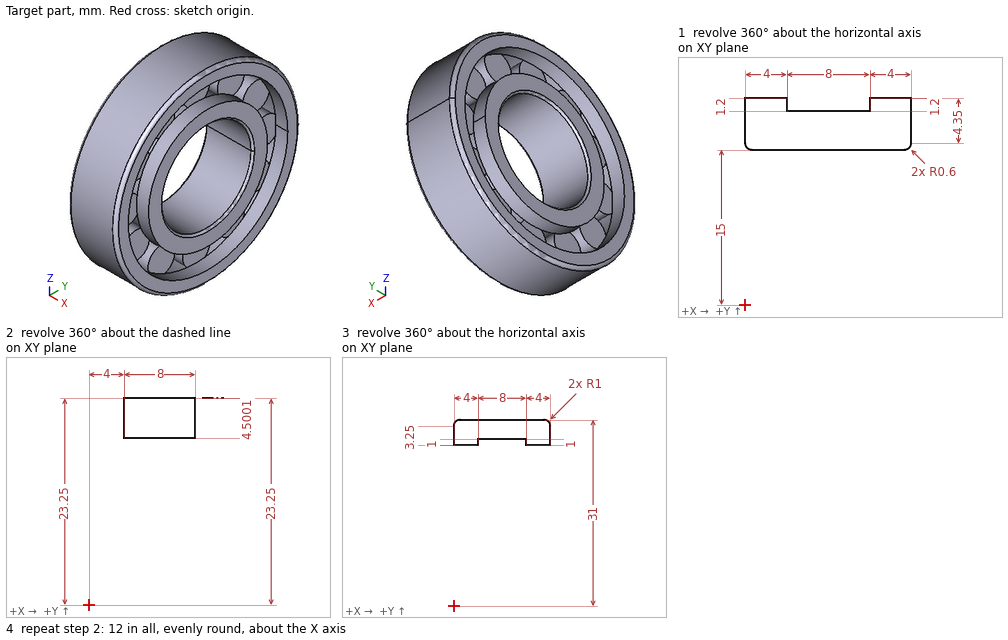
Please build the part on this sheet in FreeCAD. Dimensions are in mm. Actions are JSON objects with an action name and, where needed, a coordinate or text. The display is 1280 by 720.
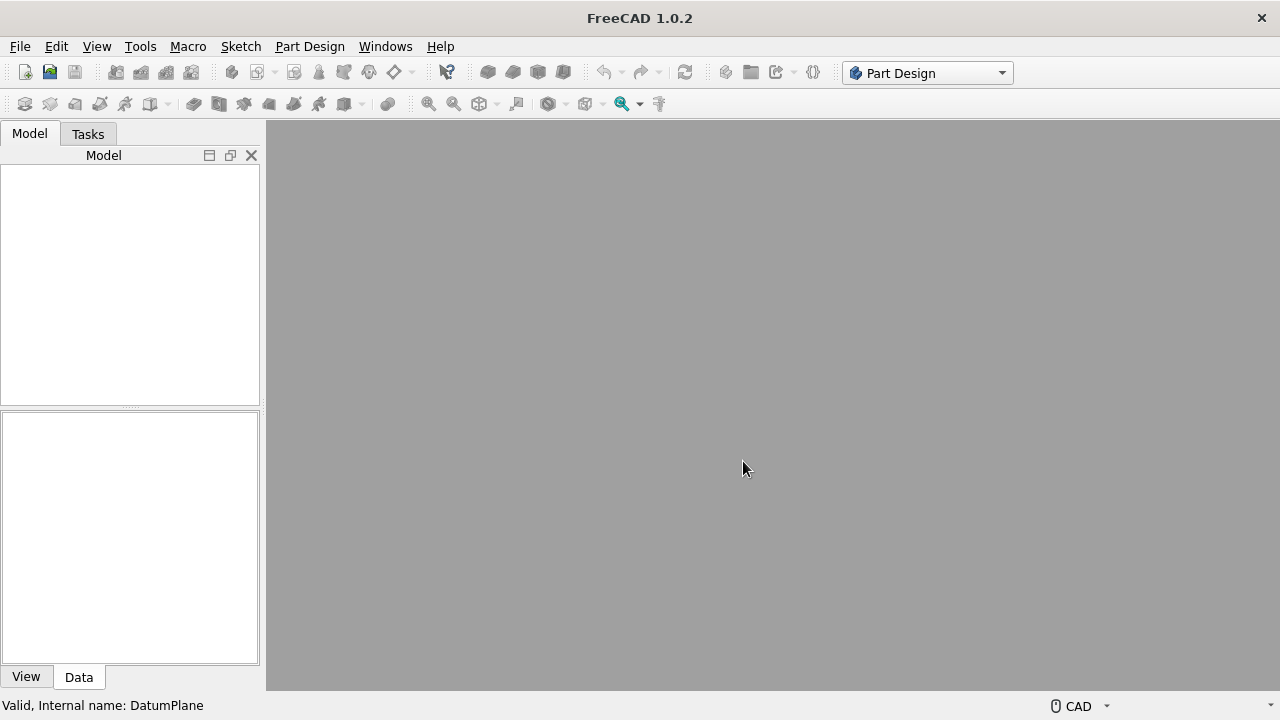
{"action": "left_click", "coordinate": [25, 72]}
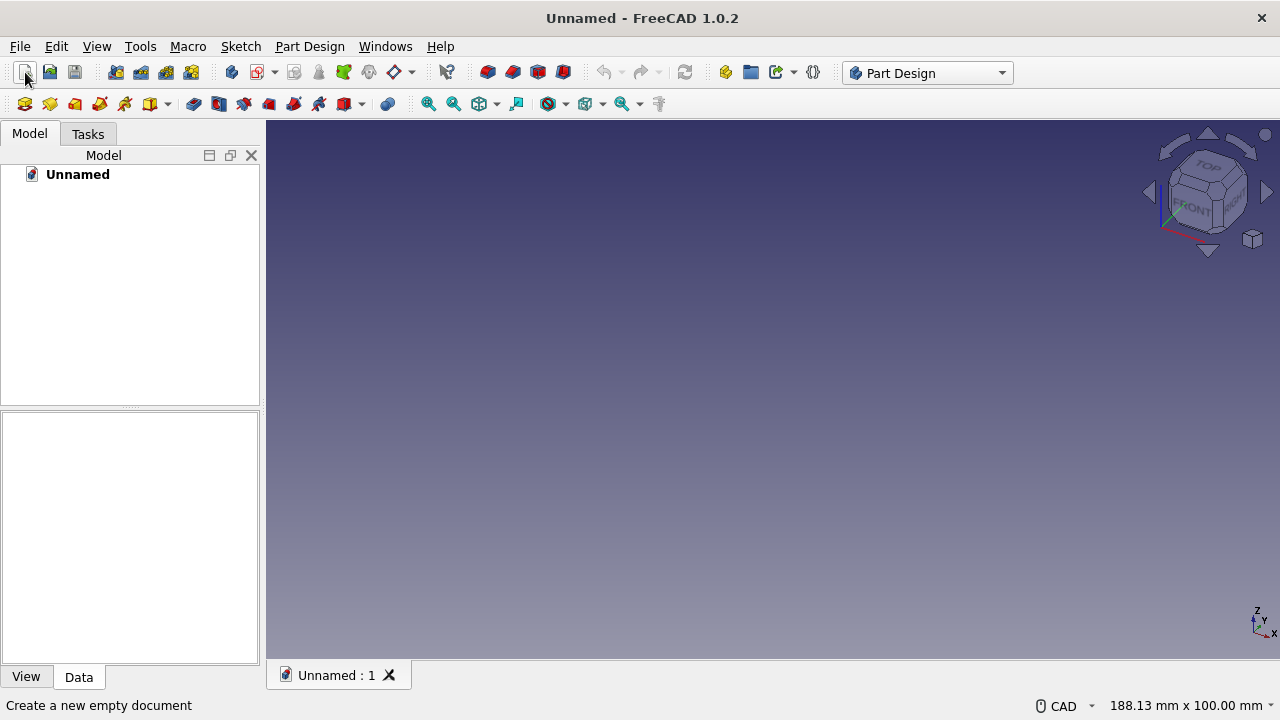
{"action": "left_click", "coordinate": [256, 72]}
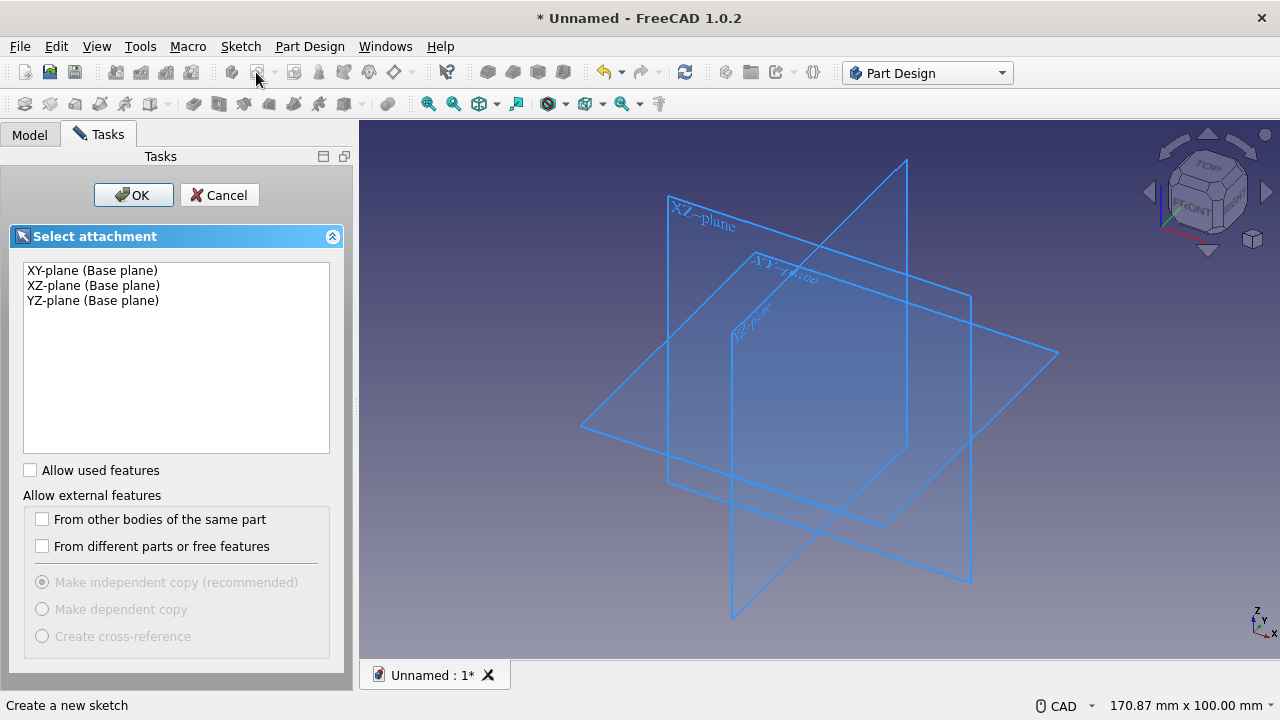
{"action": "left_click", "coordinate": [84, 270]}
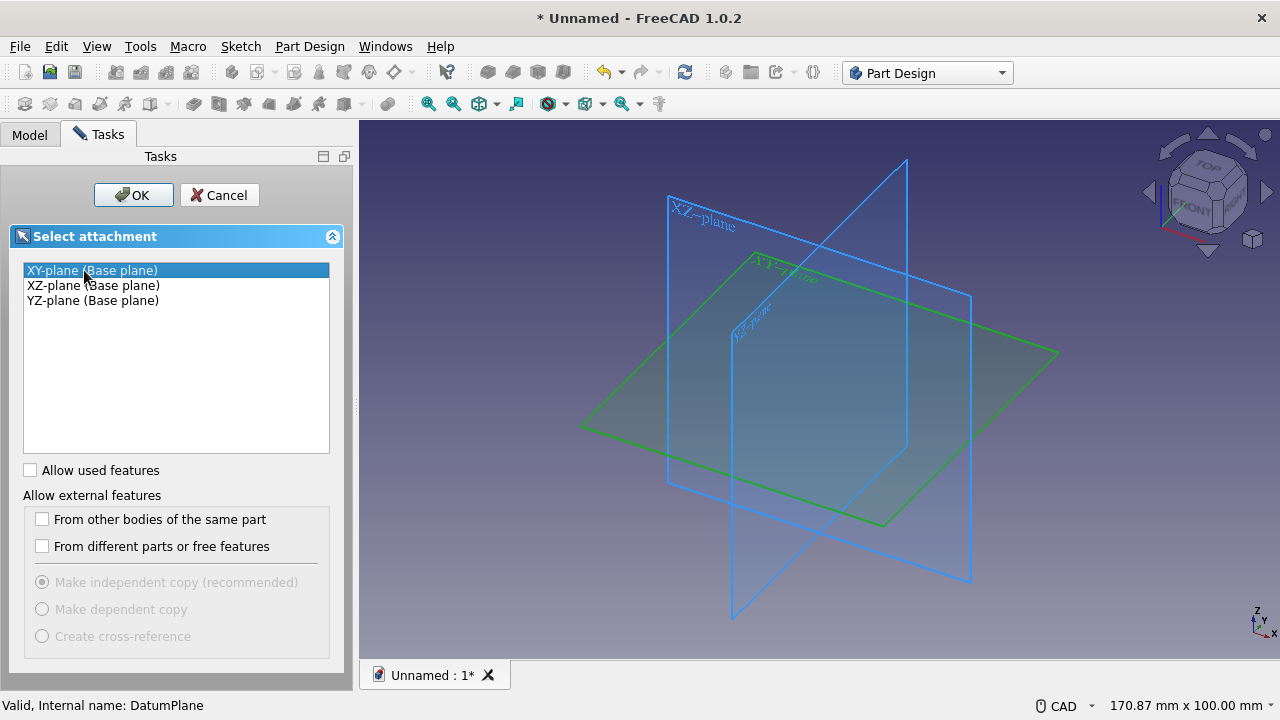
{"action": "left_click", "coordinate": [134, 195]}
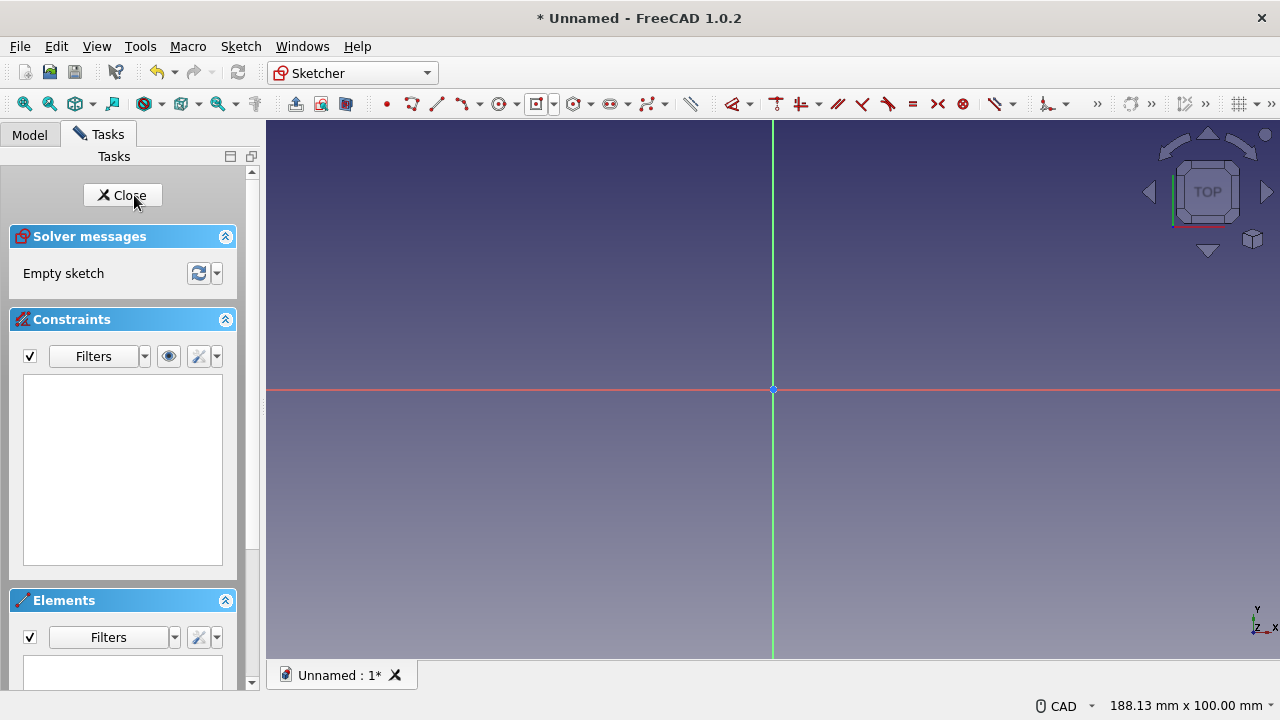
{"action": "scroll", "coordinate": [864, 313], "scroll_direction": "up", "scroll_amount": 6}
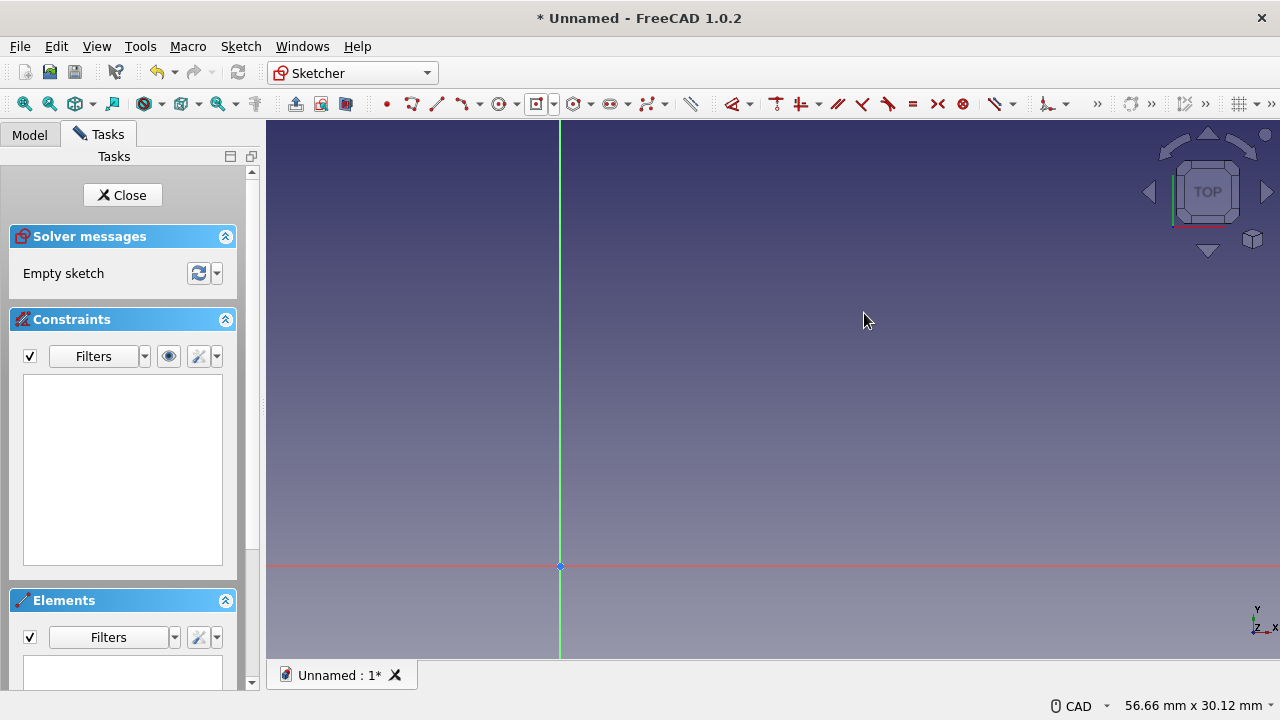
{"action": "key", "text": "g l"}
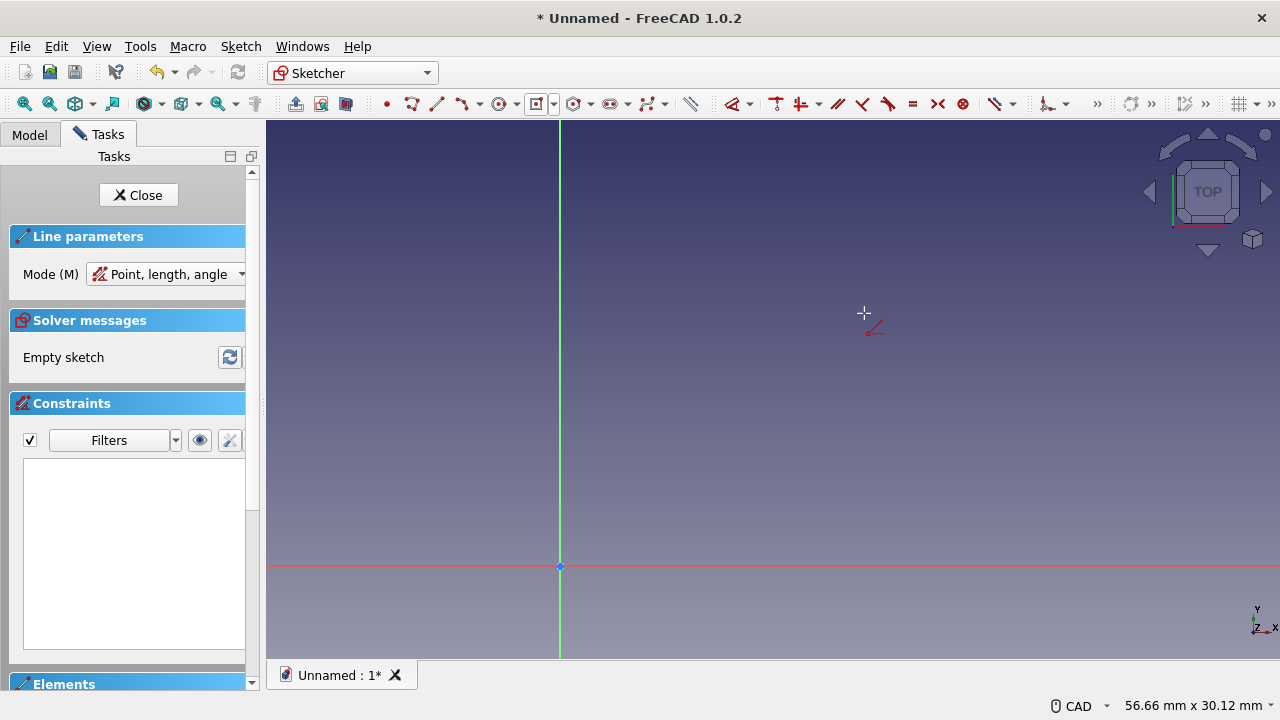
{"action": "scroll", "coordinate": [571, 298], "scroll_direction": "up", "scroll_amount": 2}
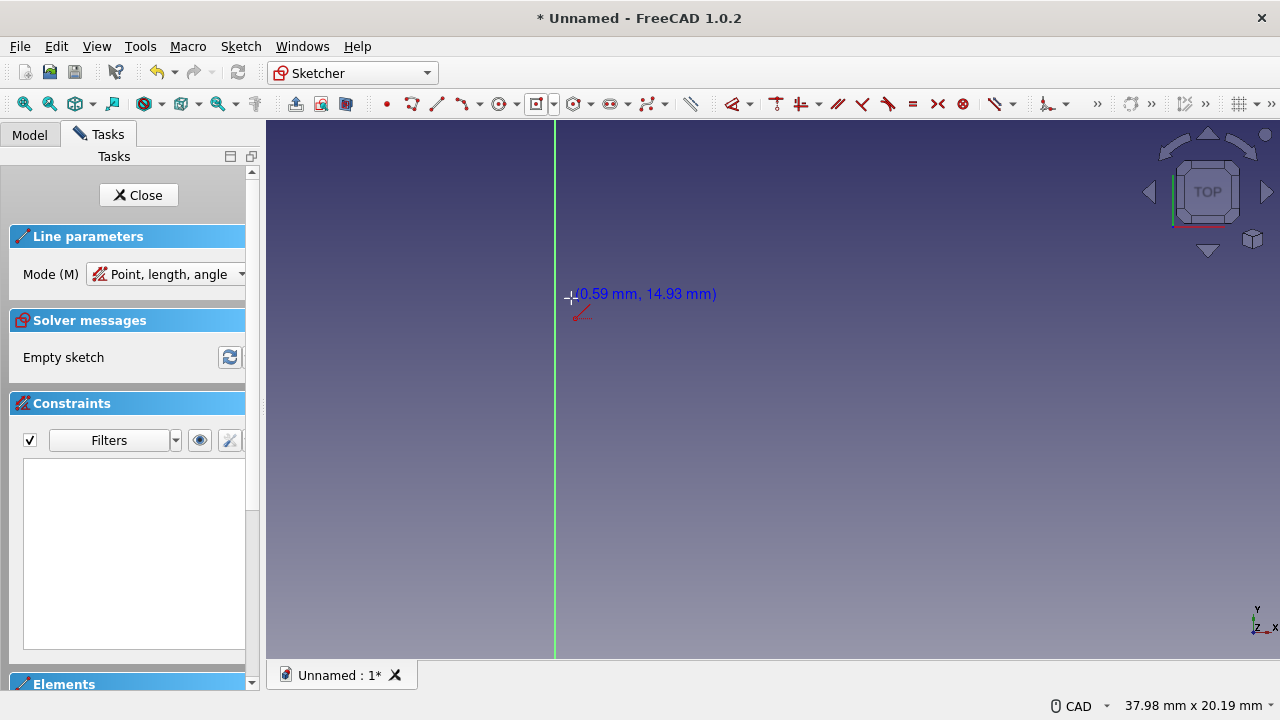
{"action": "left_click", "coordinate": [571, 297]}
{"action": "left_click", "coordinate": [966, 297]}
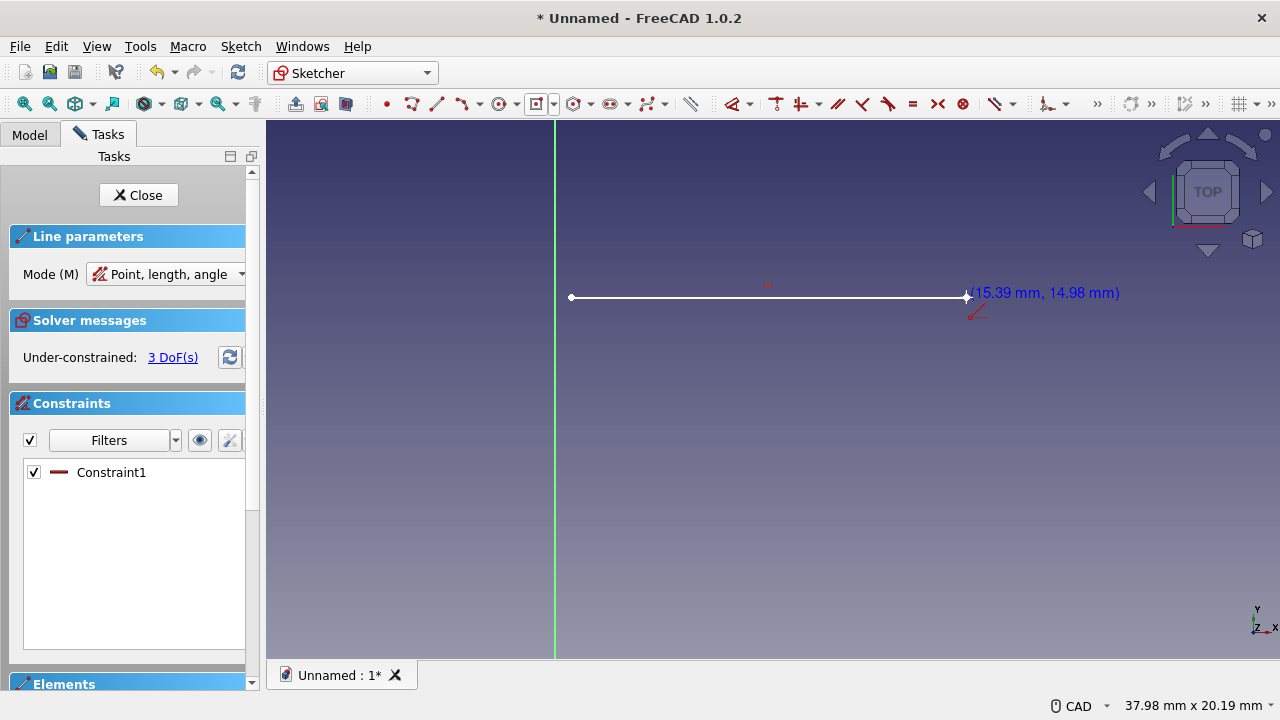
{"action": "left_click", "coordinate": [412, 104]}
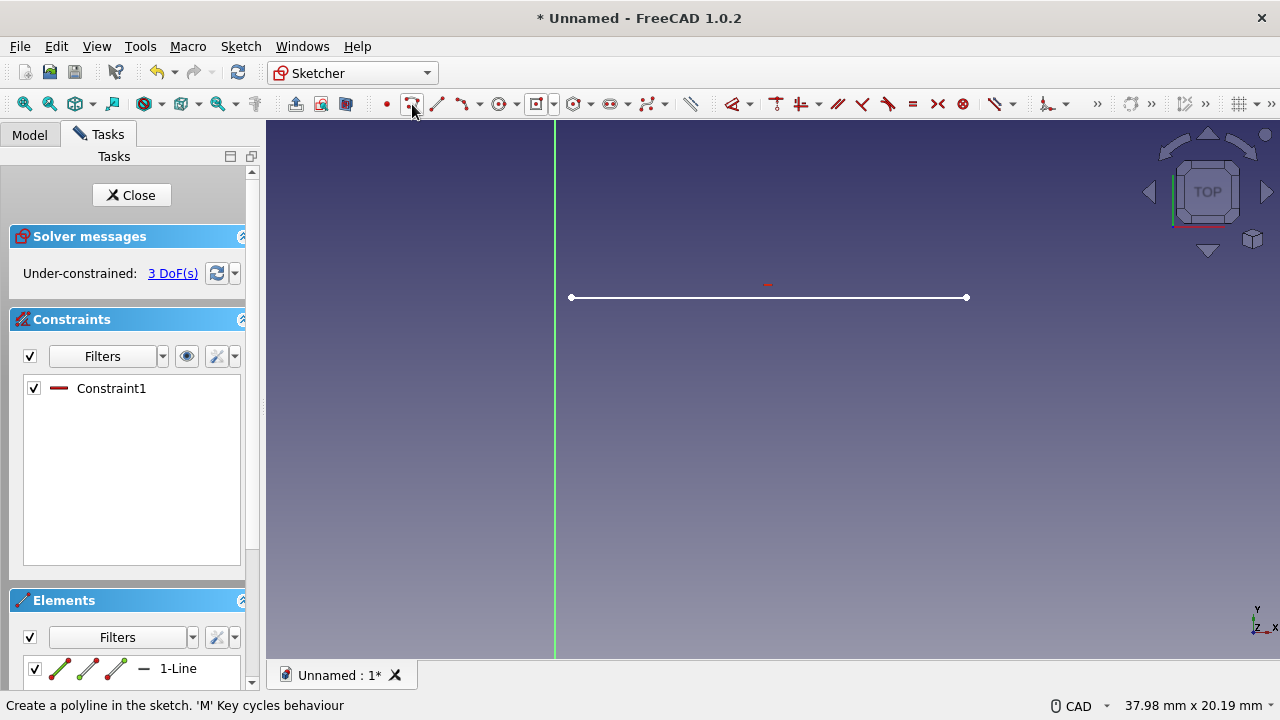
{"action": "left_click", "coordinate": [982, 281]}
{"action": "left_click", "coordinate": [982, 165]}
{"action": "left_click", "coordinate": [876, 165]}
{"action": "left_click", "coordinate": [876, 197]}
{"action": "left_click", "coordinate": [662, 197]}
{"action": "left_click", "coordinate": [662, 165]}
{"action": "left_click", "coordinate": [555, 165]}
{"action": "left_click", "coordinate": [564, 281]}
{"action": "right_click", "coordinate": [564, 281]}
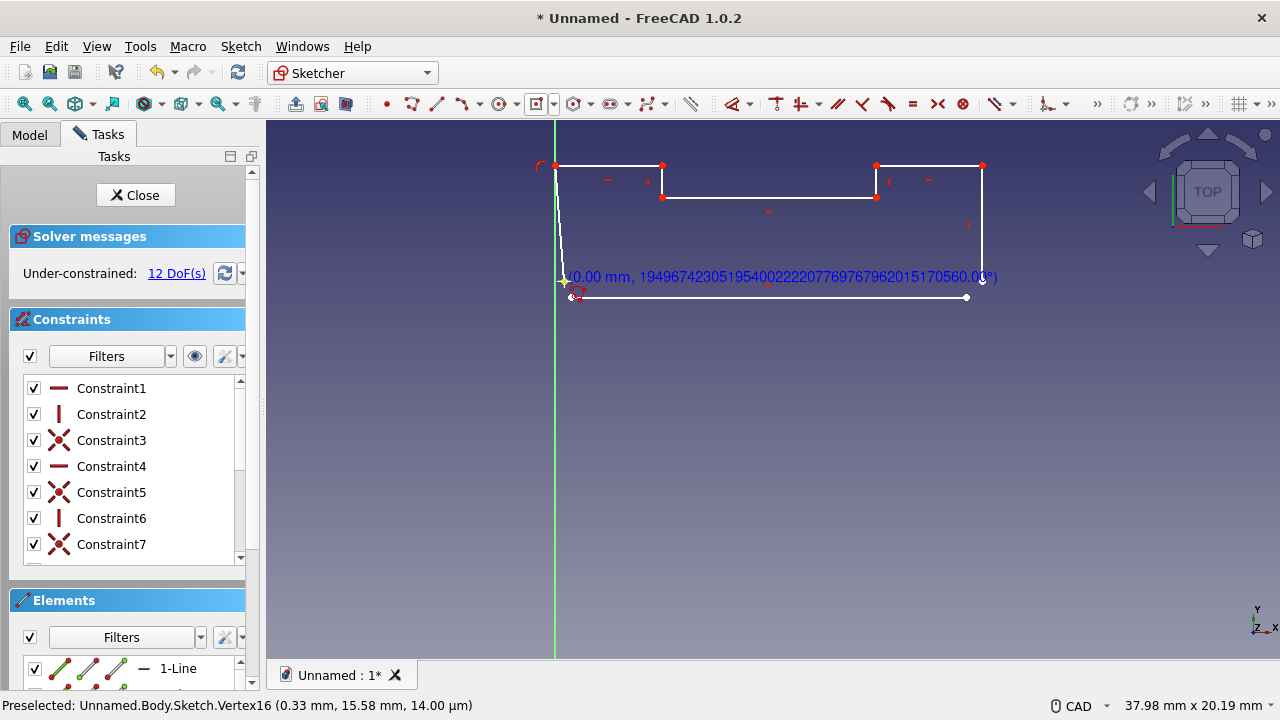
{"action": "key", "text": "g 3 a"}